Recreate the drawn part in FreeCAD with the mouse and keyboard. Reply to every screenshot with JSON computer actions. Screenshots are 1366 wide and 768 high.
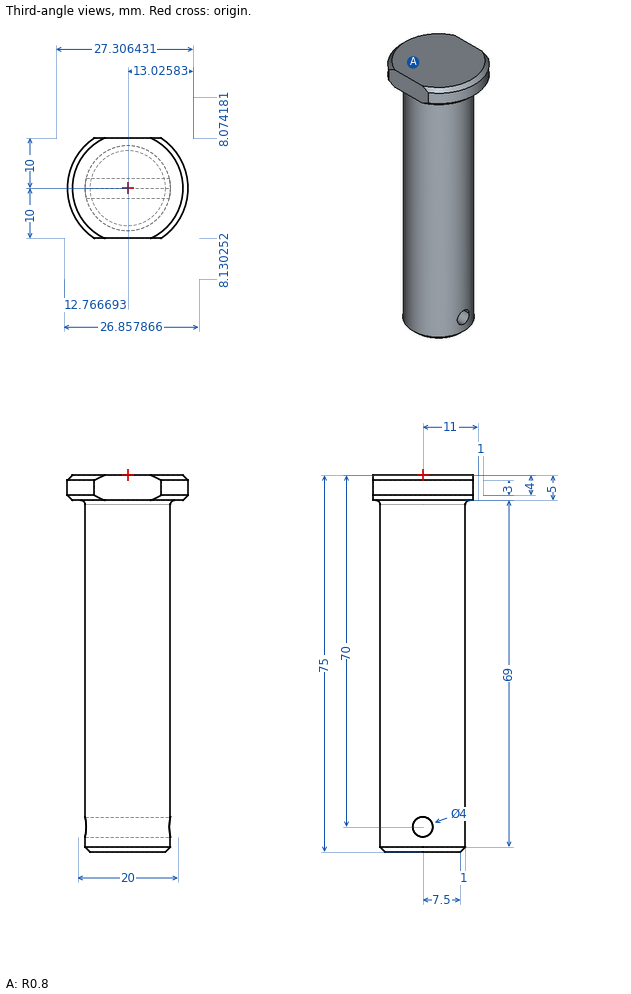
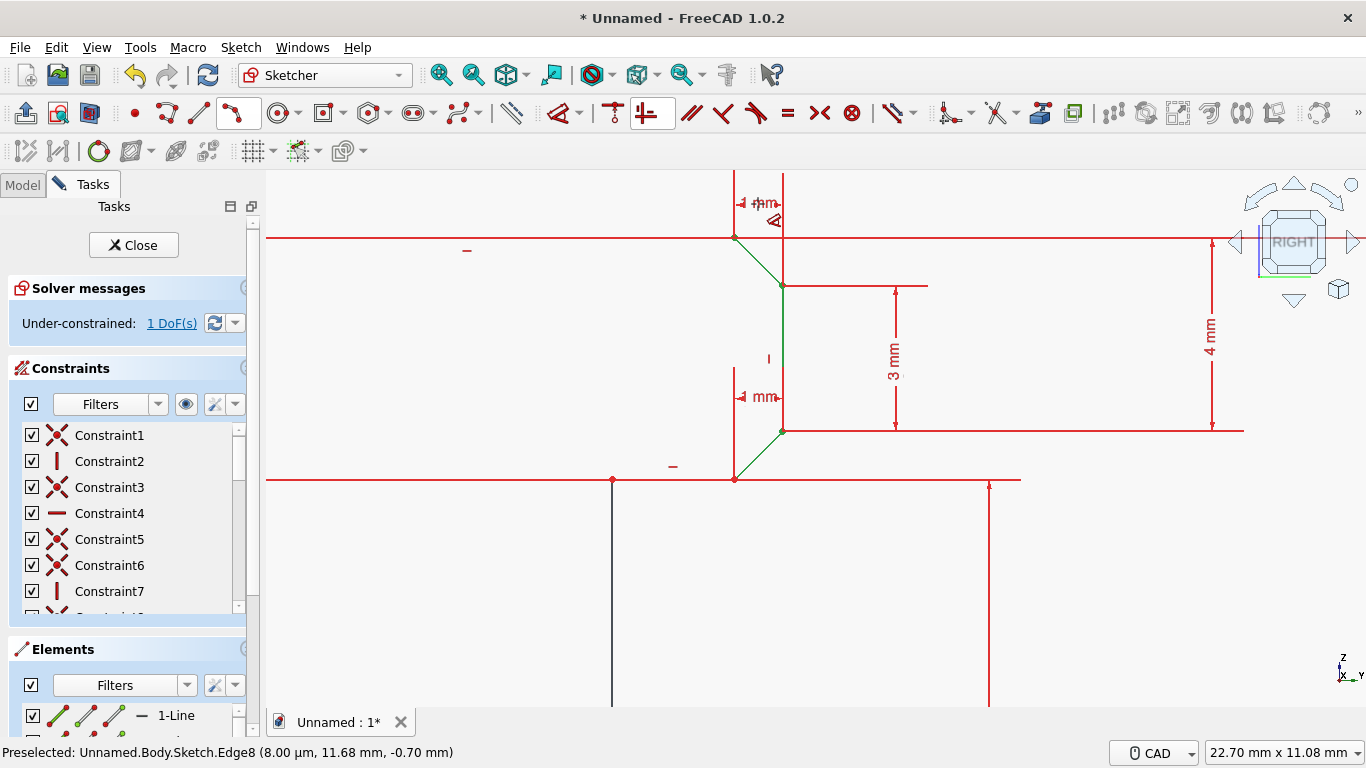
{"action": "scroll", "coordinate": [773, 277], "scroll_direction": "down", "scroll_amount": 12}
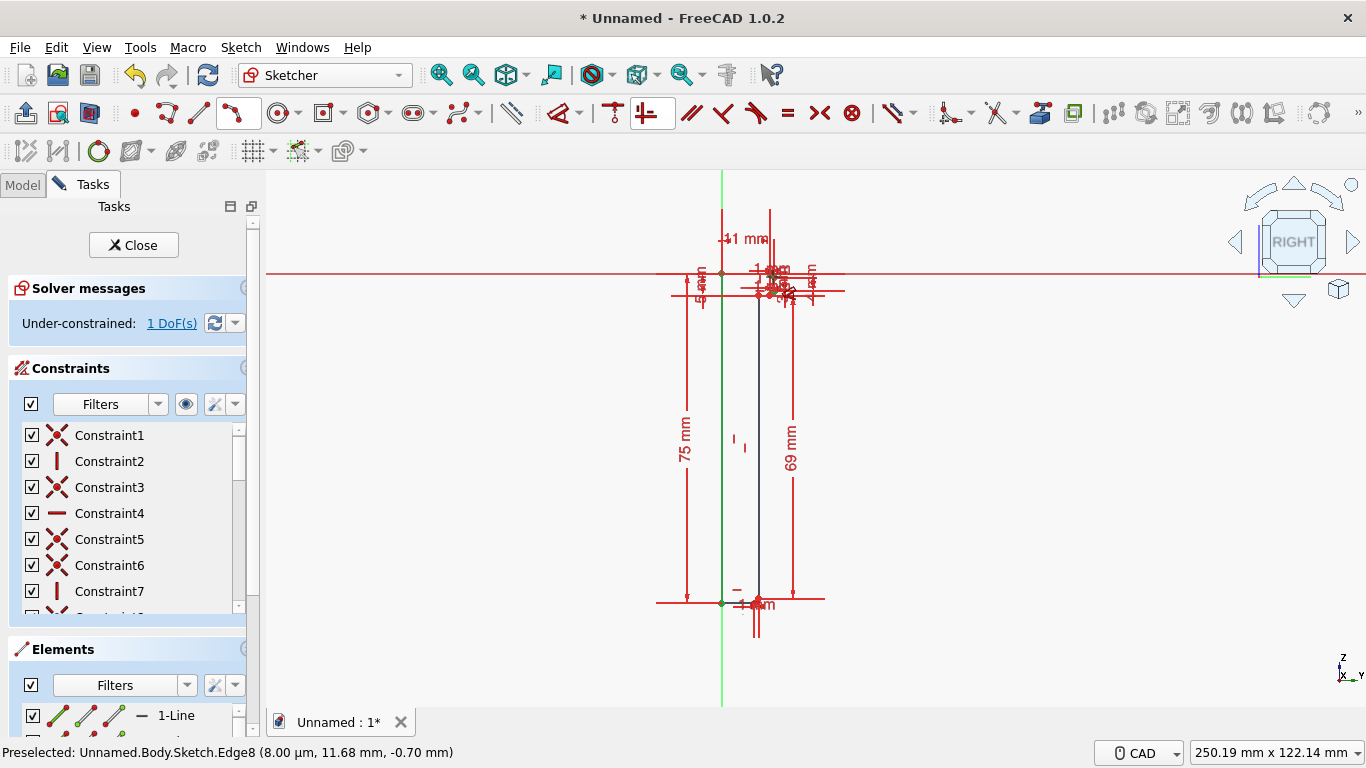
{"action": "scroll", "coordinate": [731, 603], "scroll_direction": "up", "scroll_amount": 2}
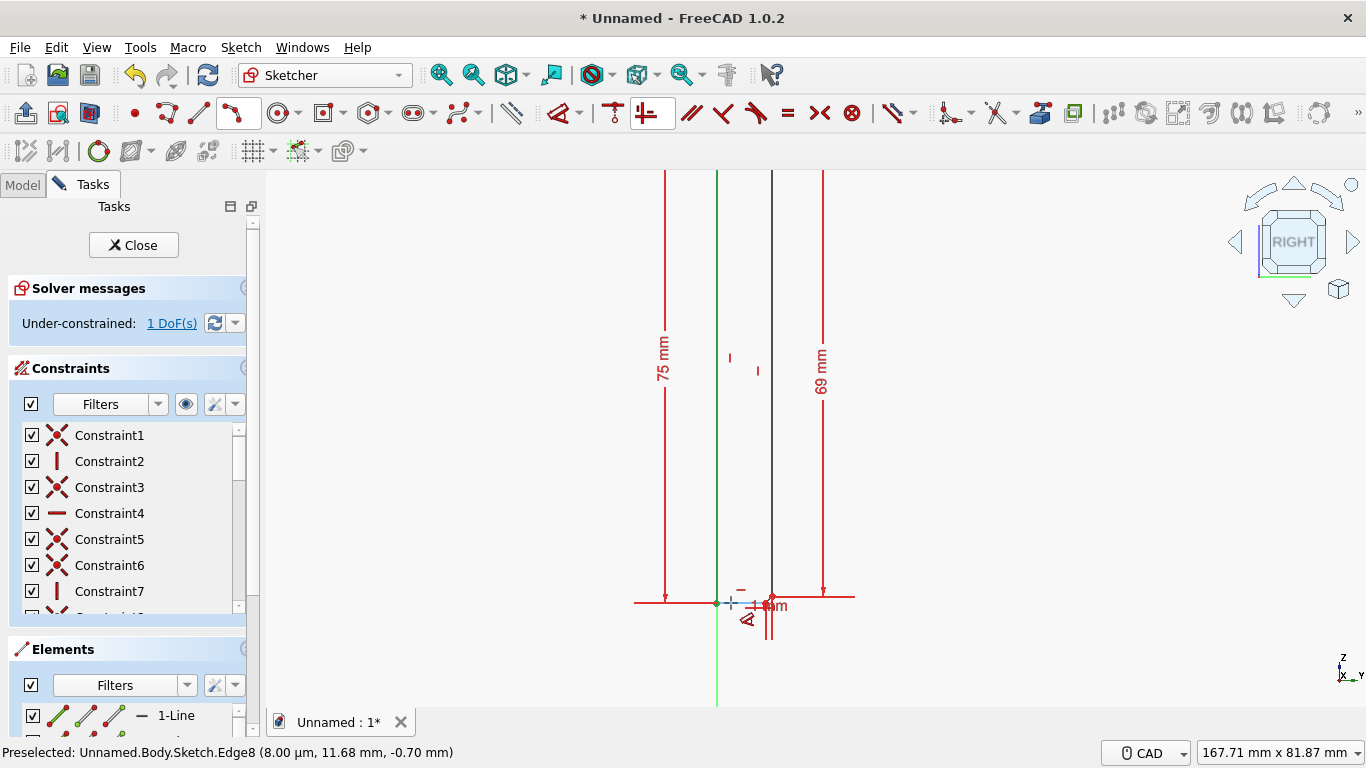
{"action": "left_click", "coordinate": [731, 603]}
{"action": "left_click", "coordinate": [741, 637]}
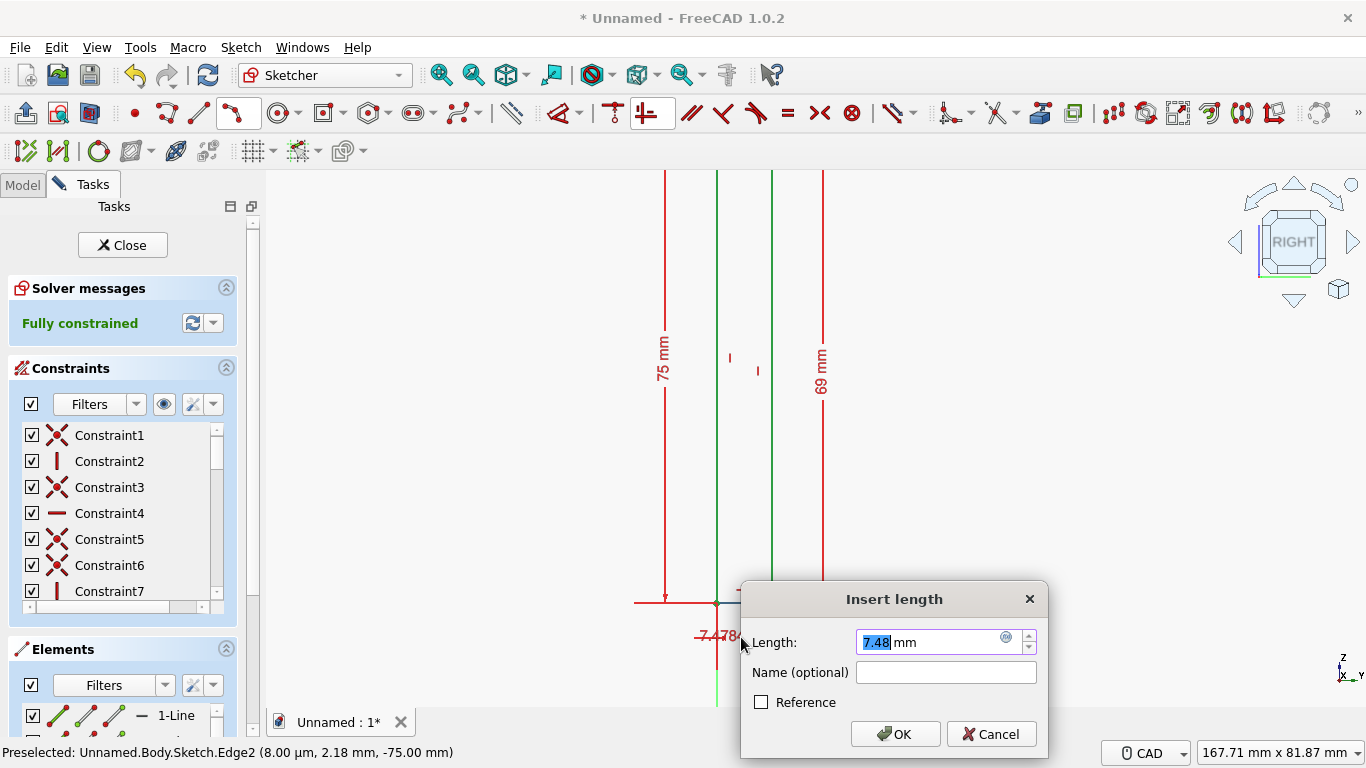
{"action": "type", "text": "7.5"}
{"action": "key", "text": "Return"}
{"action": "key", "text": "Escape"}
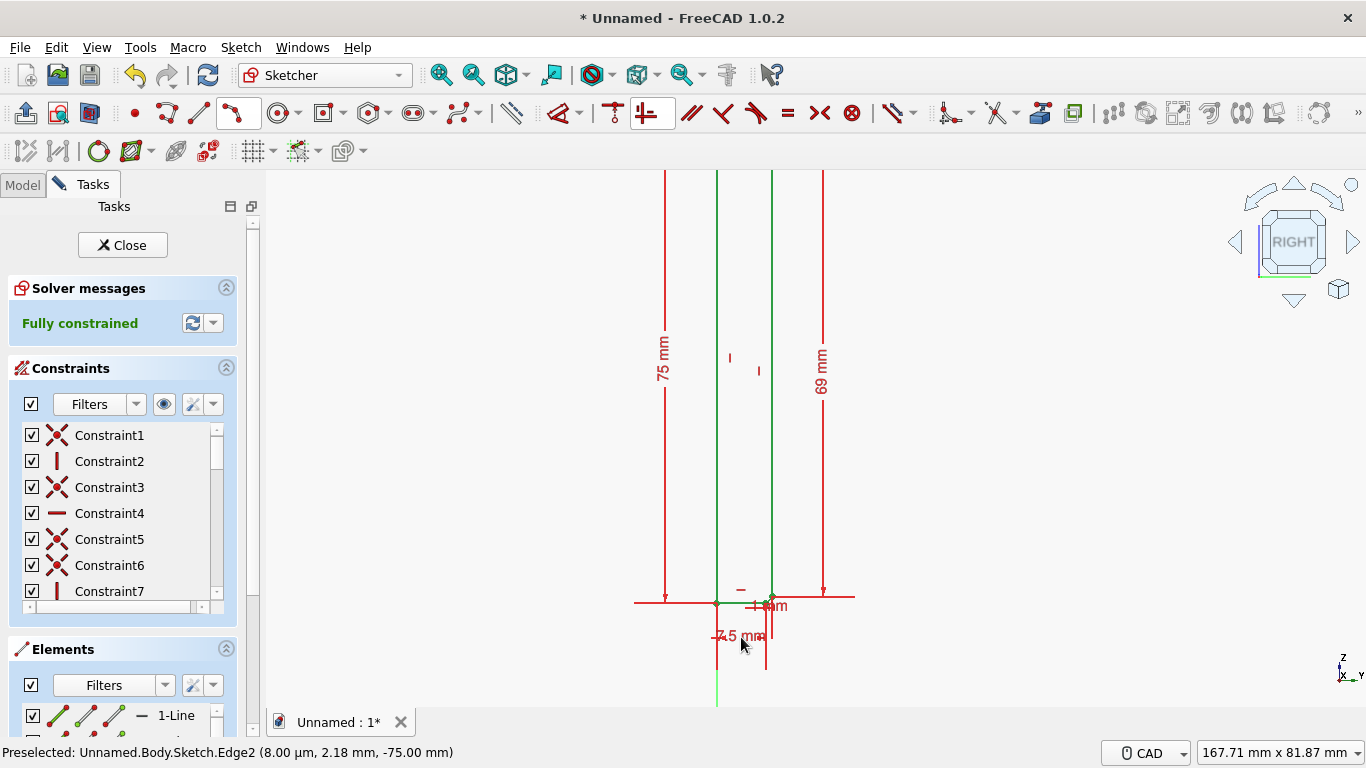
{"action": "left_click", "coordinate": [123, 245]}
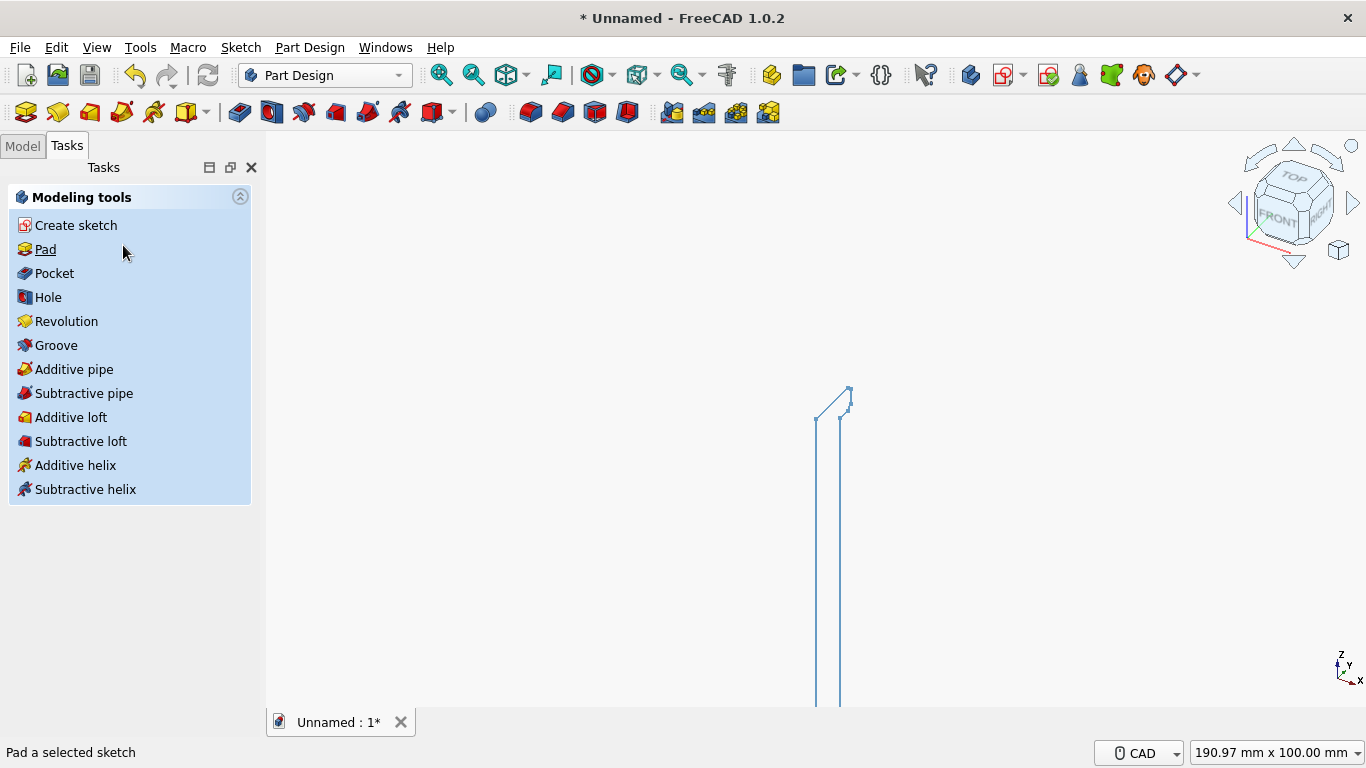
{"action": "left_click", "coordinate": [58, 112]}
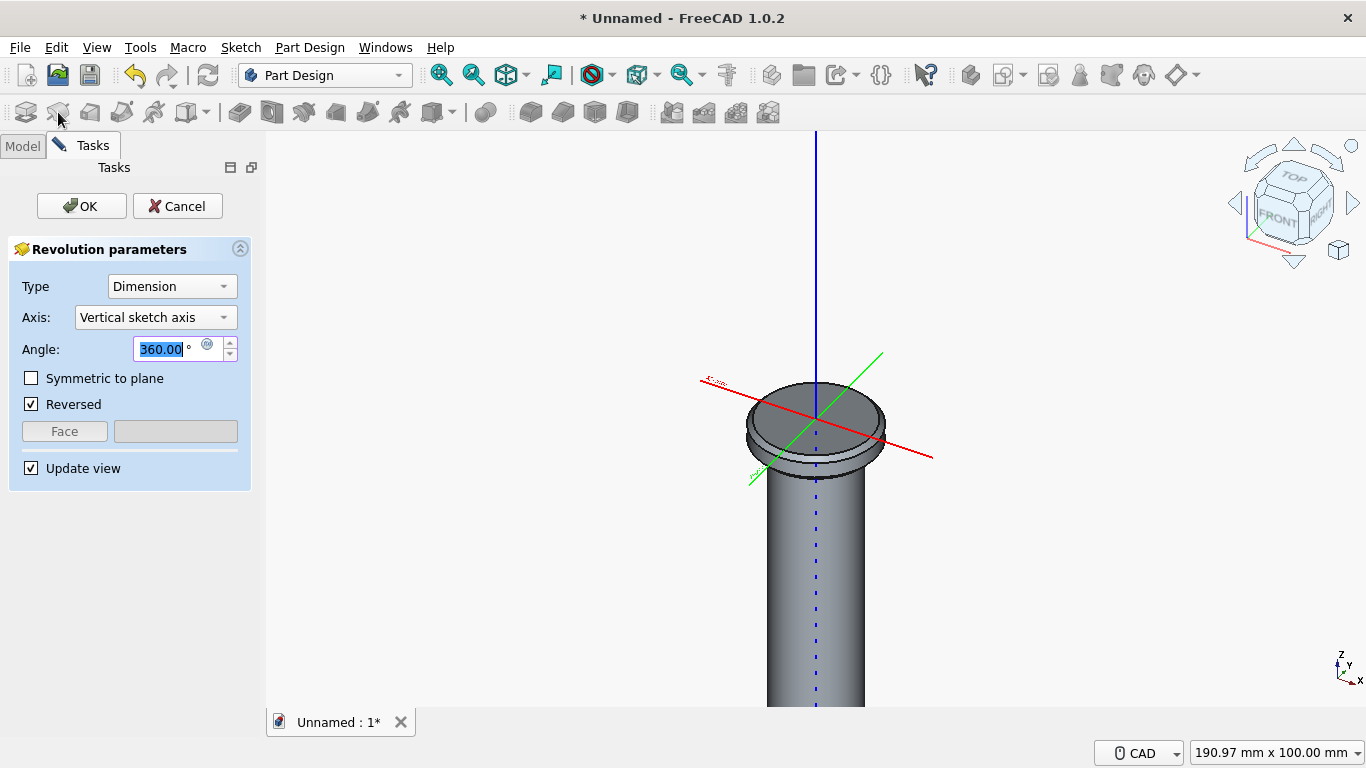
{"action": "left_click", "coordinate": [82, 206]}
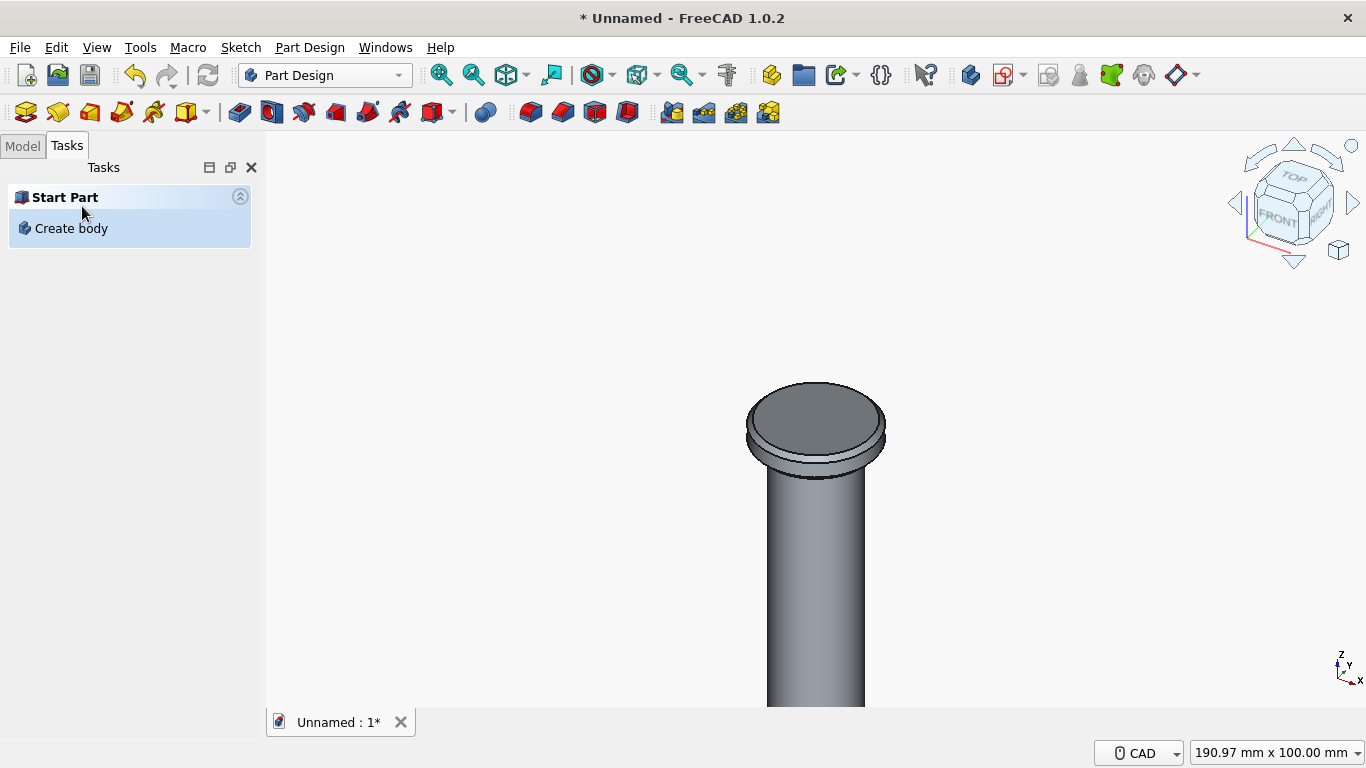
{"action": "left_click", "coordinate": [442, 76]}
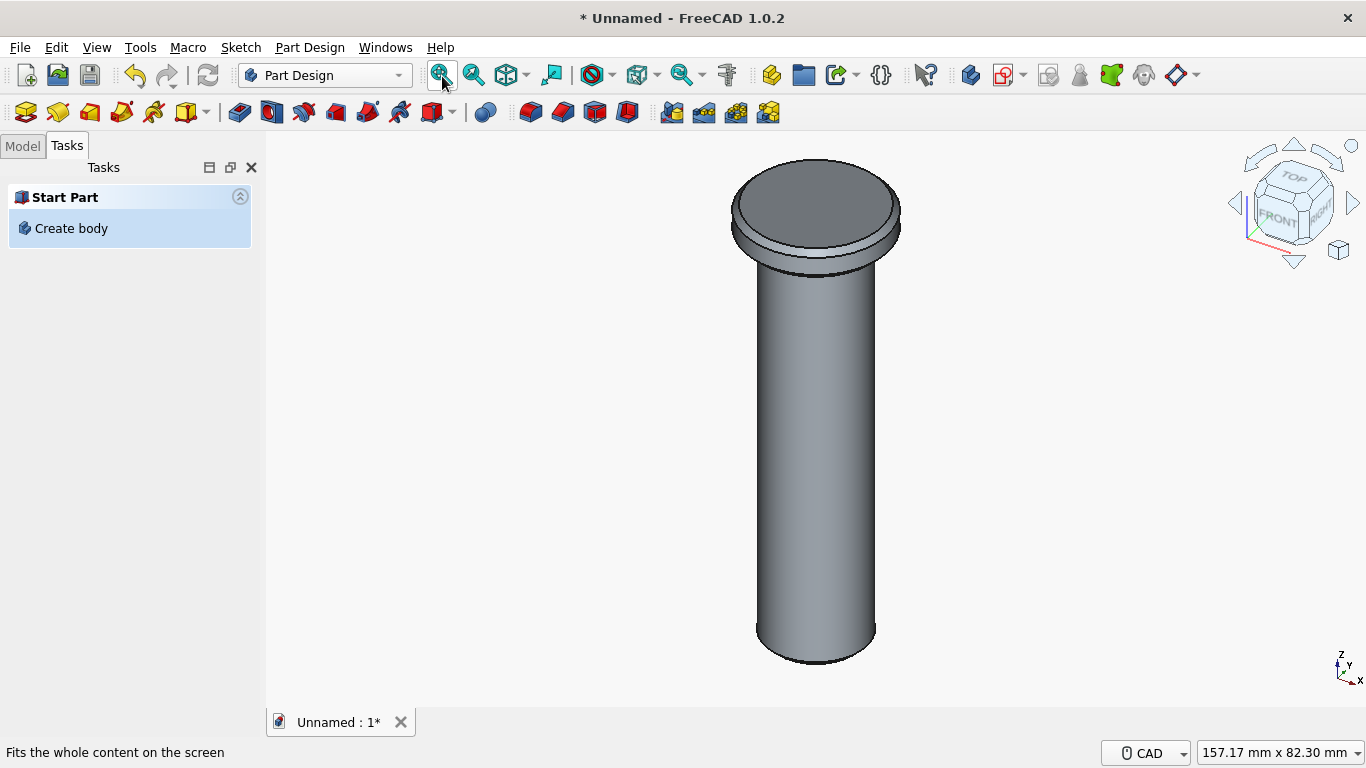
{"action": "left_click", "coordinate": [1004, 76]}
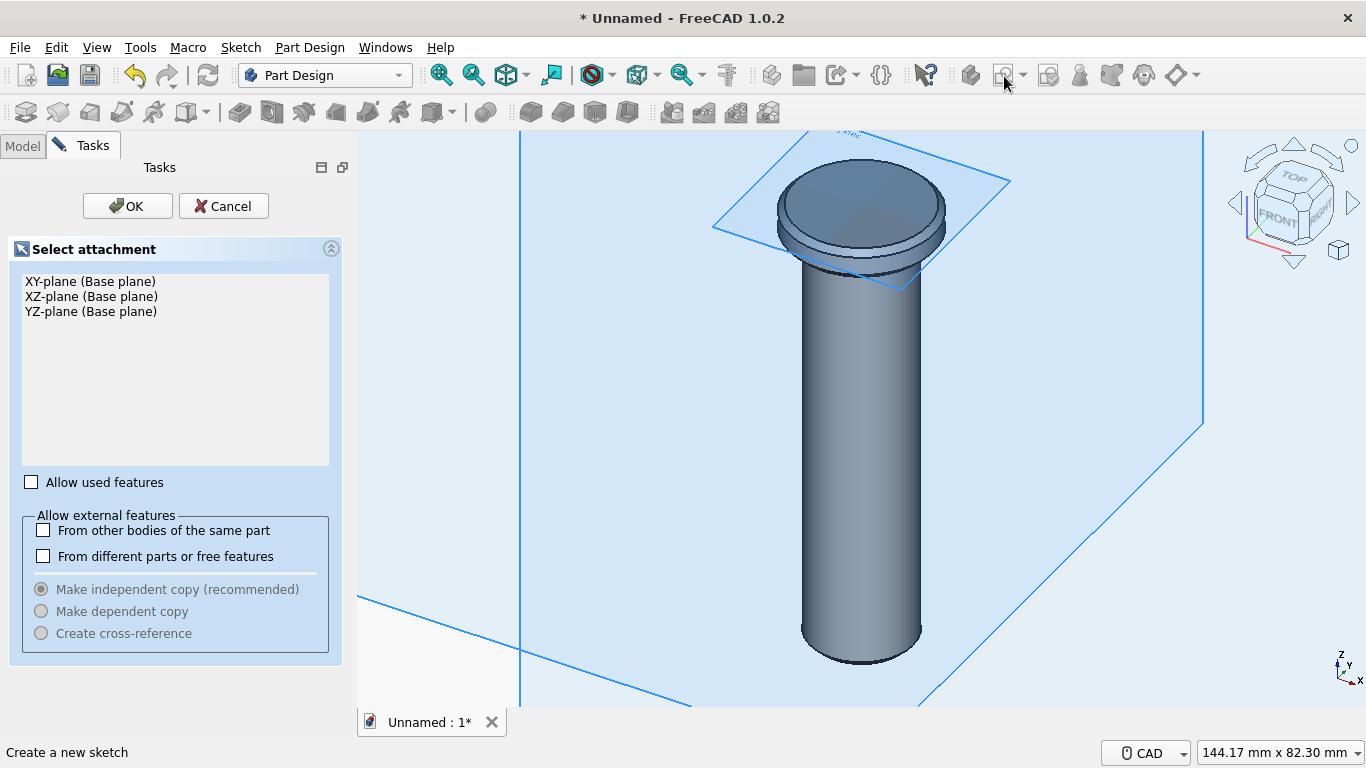
{"action": "left_click", "coordinate": [82, 312]}